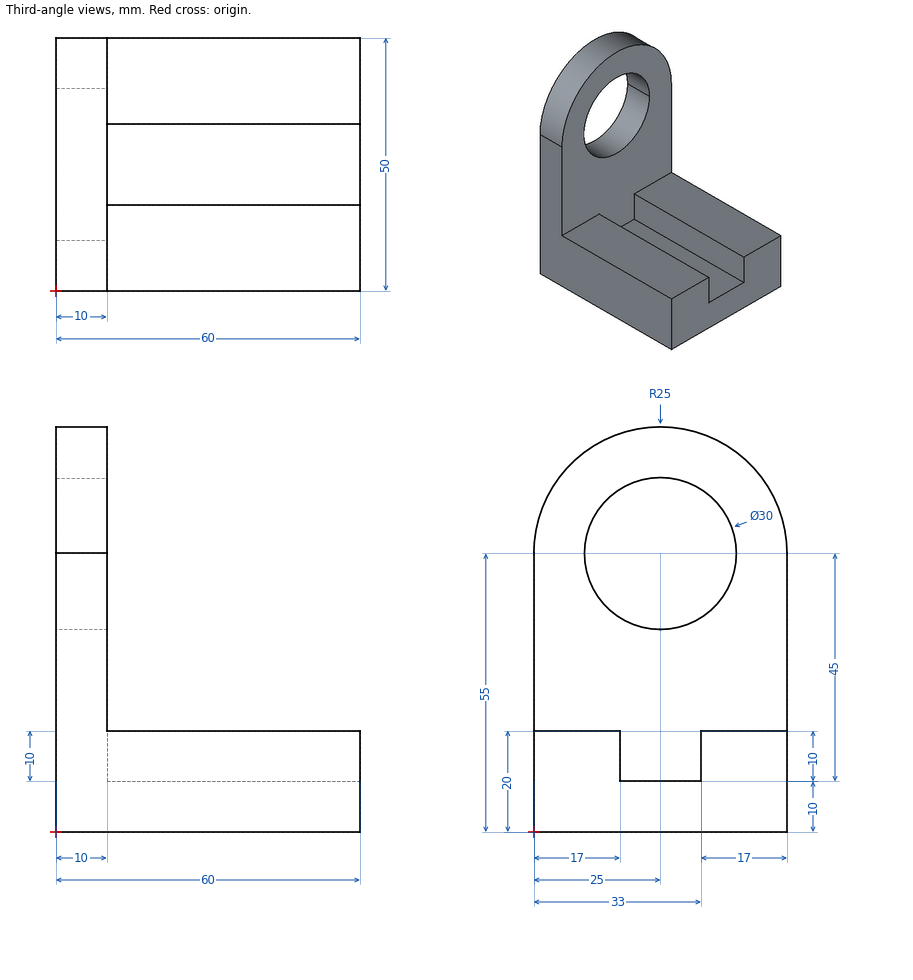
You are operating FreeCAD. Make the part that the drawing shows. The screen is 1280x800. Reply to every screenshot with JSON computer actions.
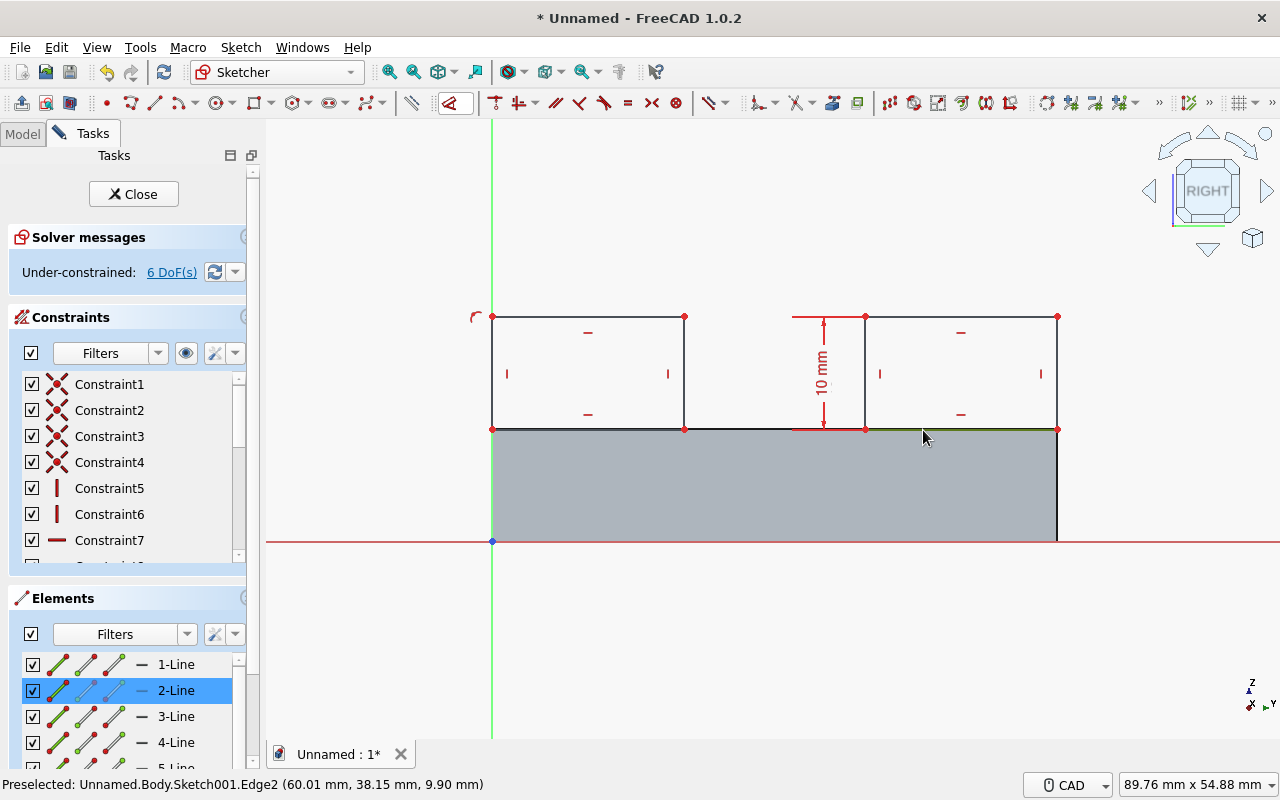
{"action": "key", "text": "l"}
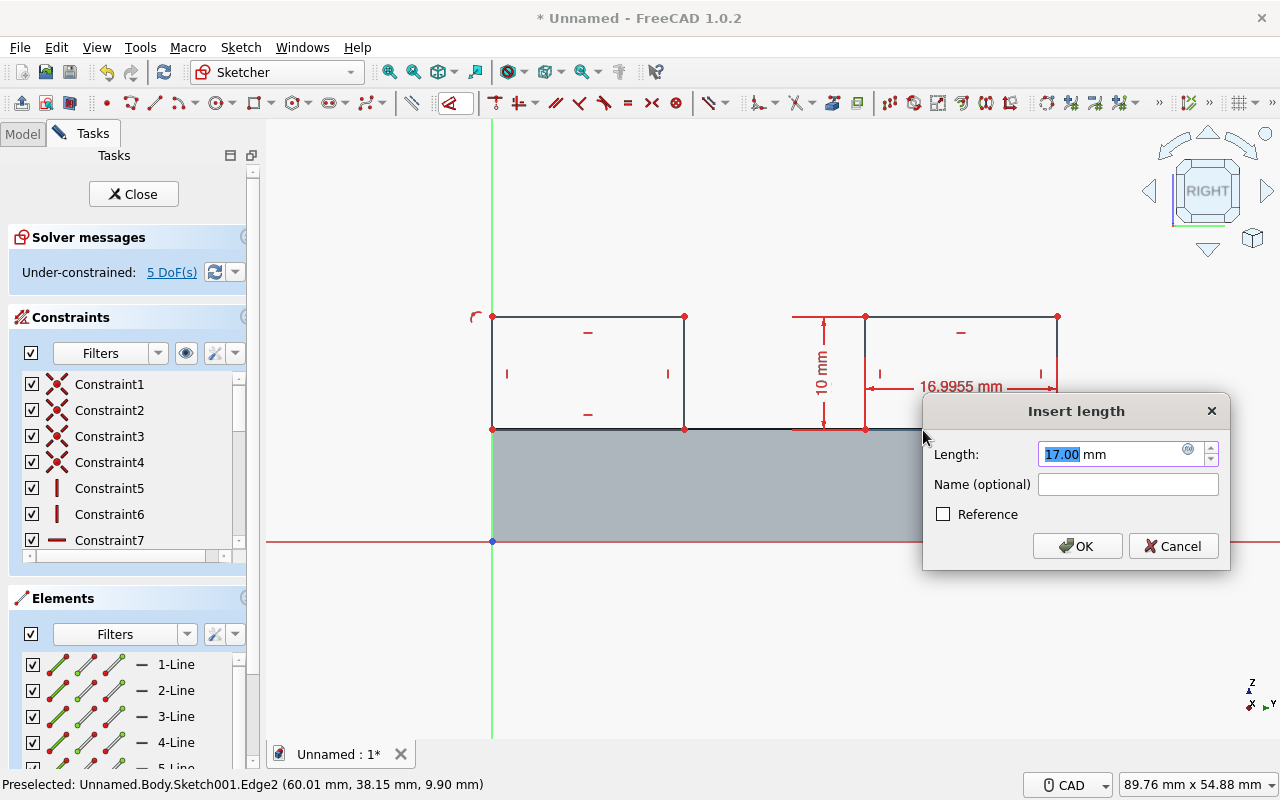
{"action": "type", "text": "17"}
{"action": "key", "text": "Return"}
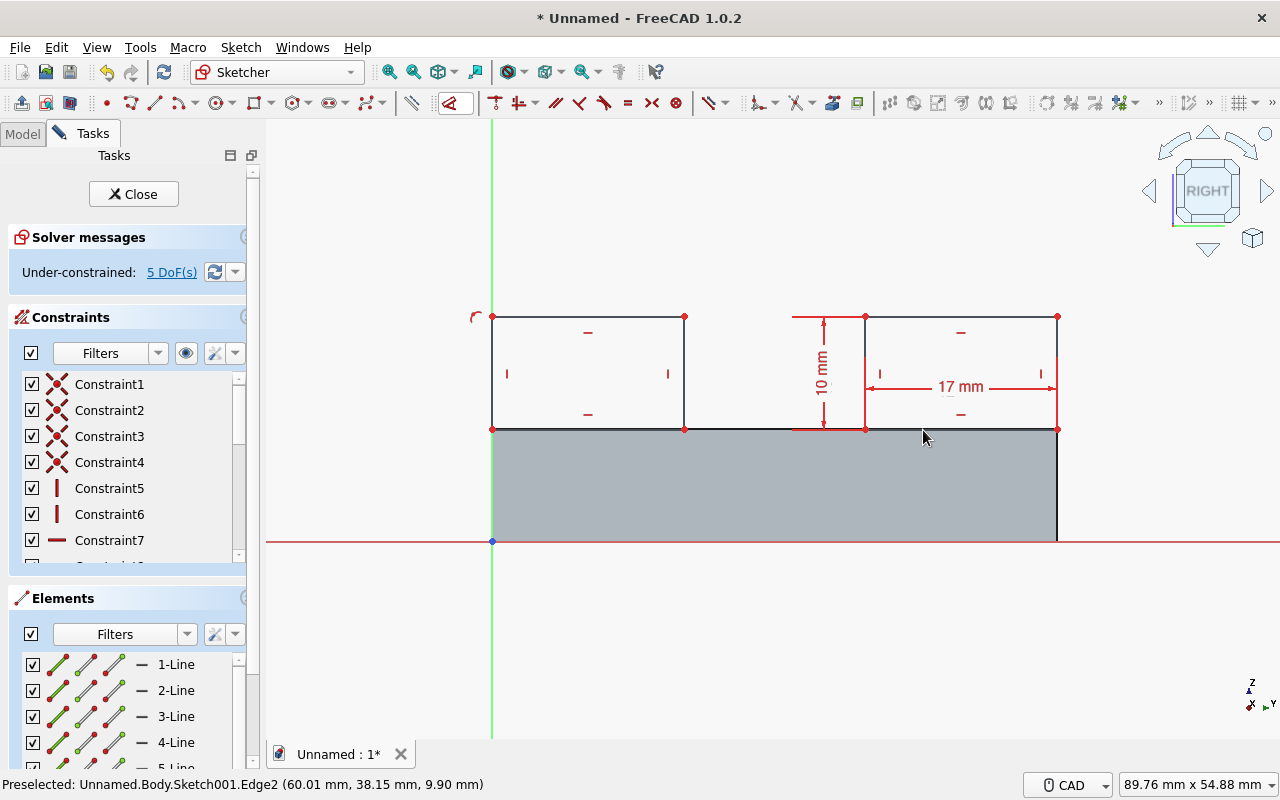
{"action": "left_click", "coordinate": [492, 351]}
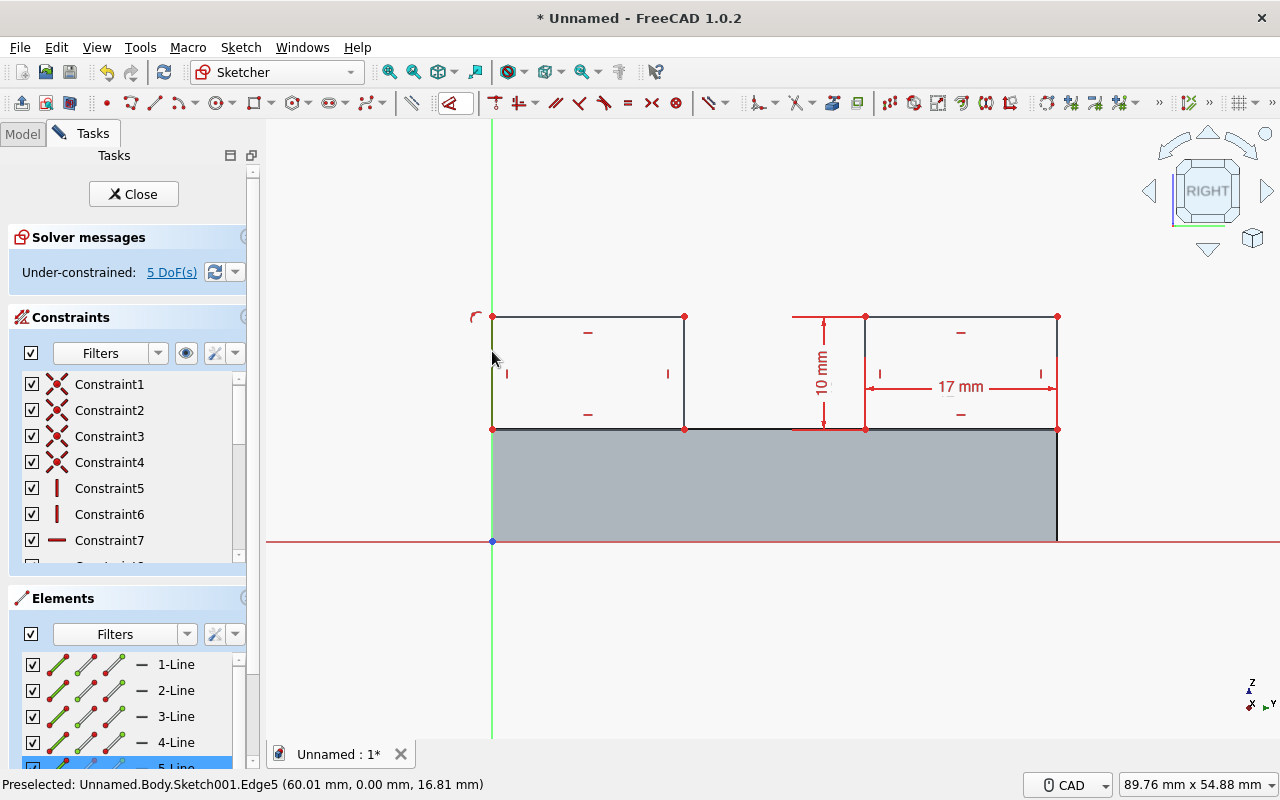
{"action": "left_click", "coordinate": [468, 104]}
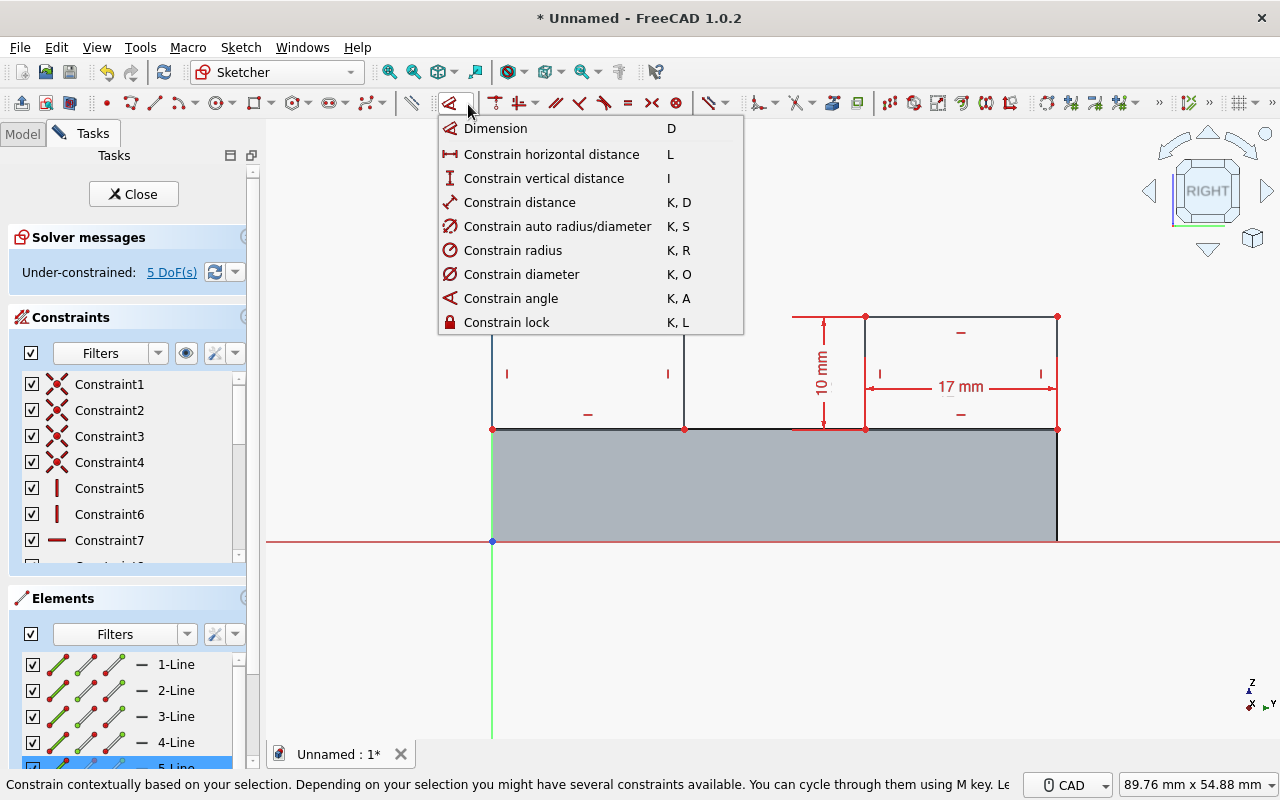
{"action": "left_click", "coordinate": [591, 178]}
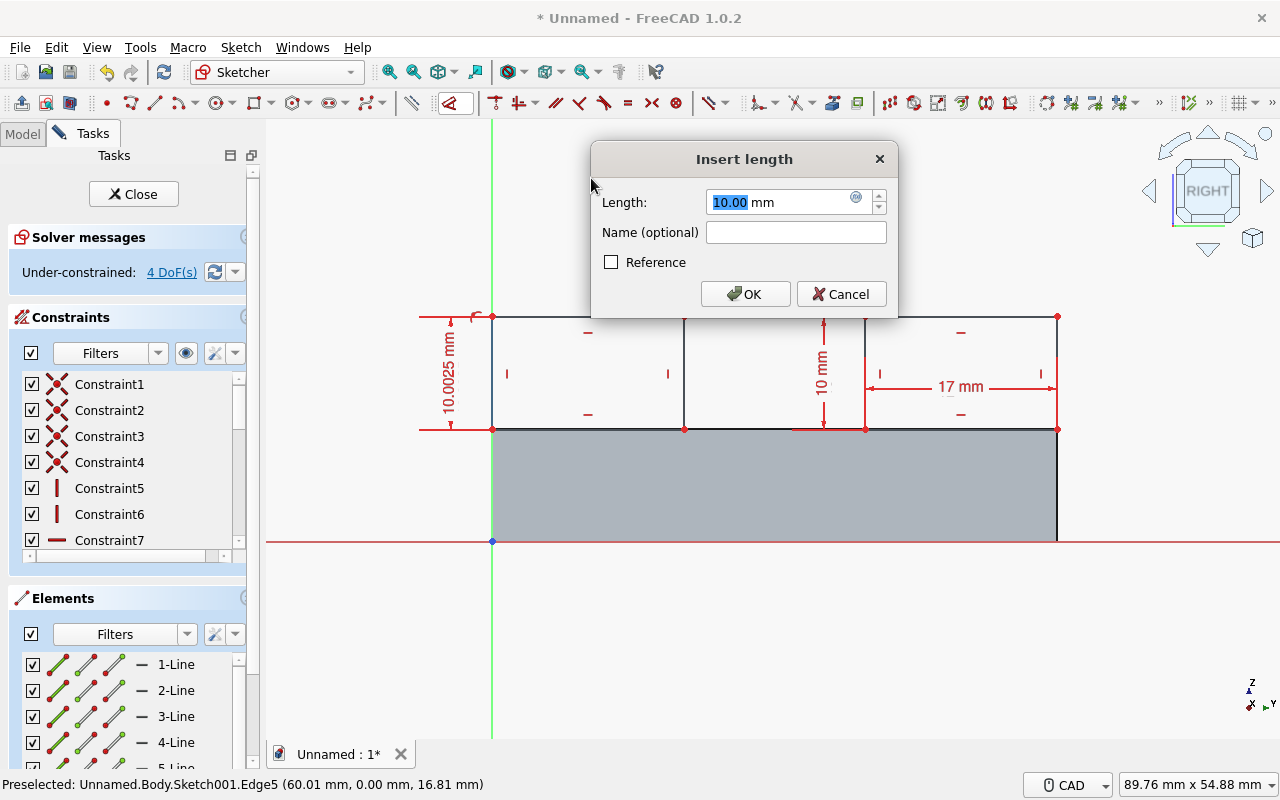
{"action": "type", "text": "10"}
{"action": "key", "text": "Return"}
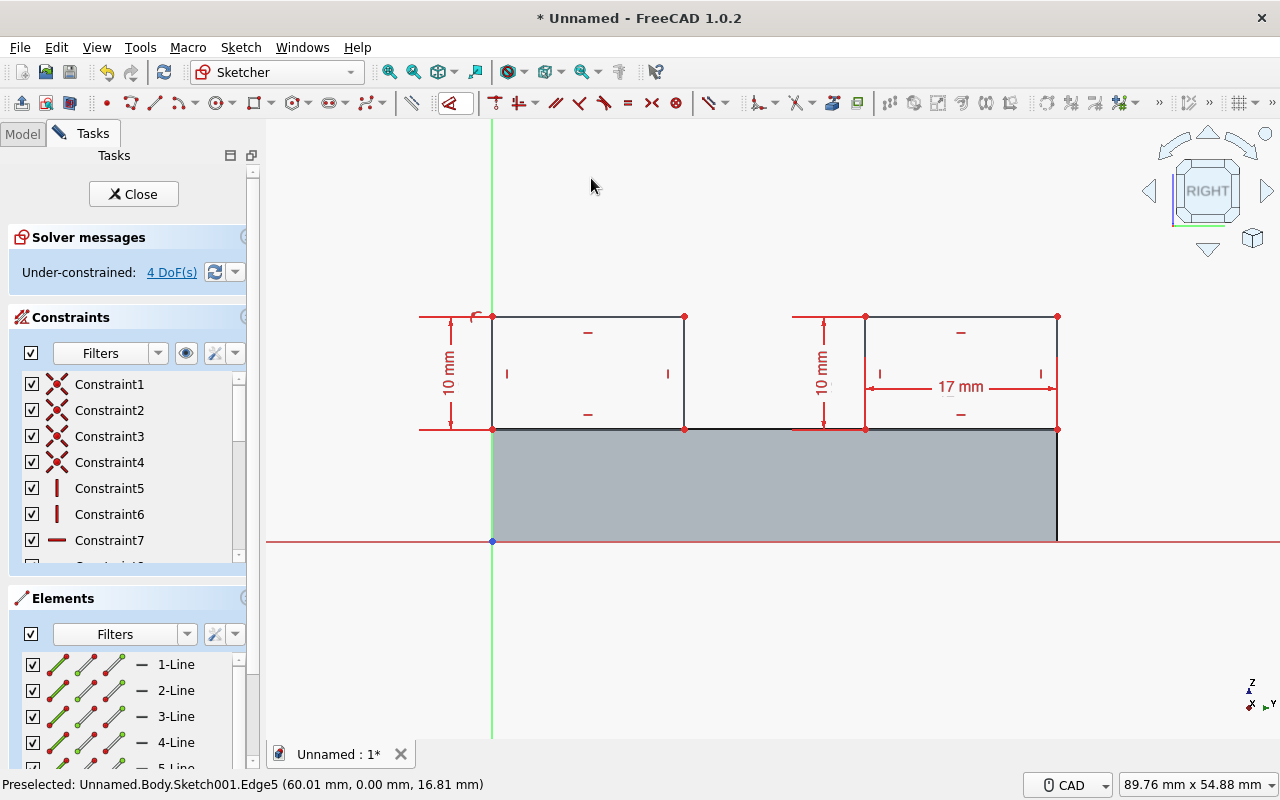
{"action": "left_click", "coordinate": [550, 430]}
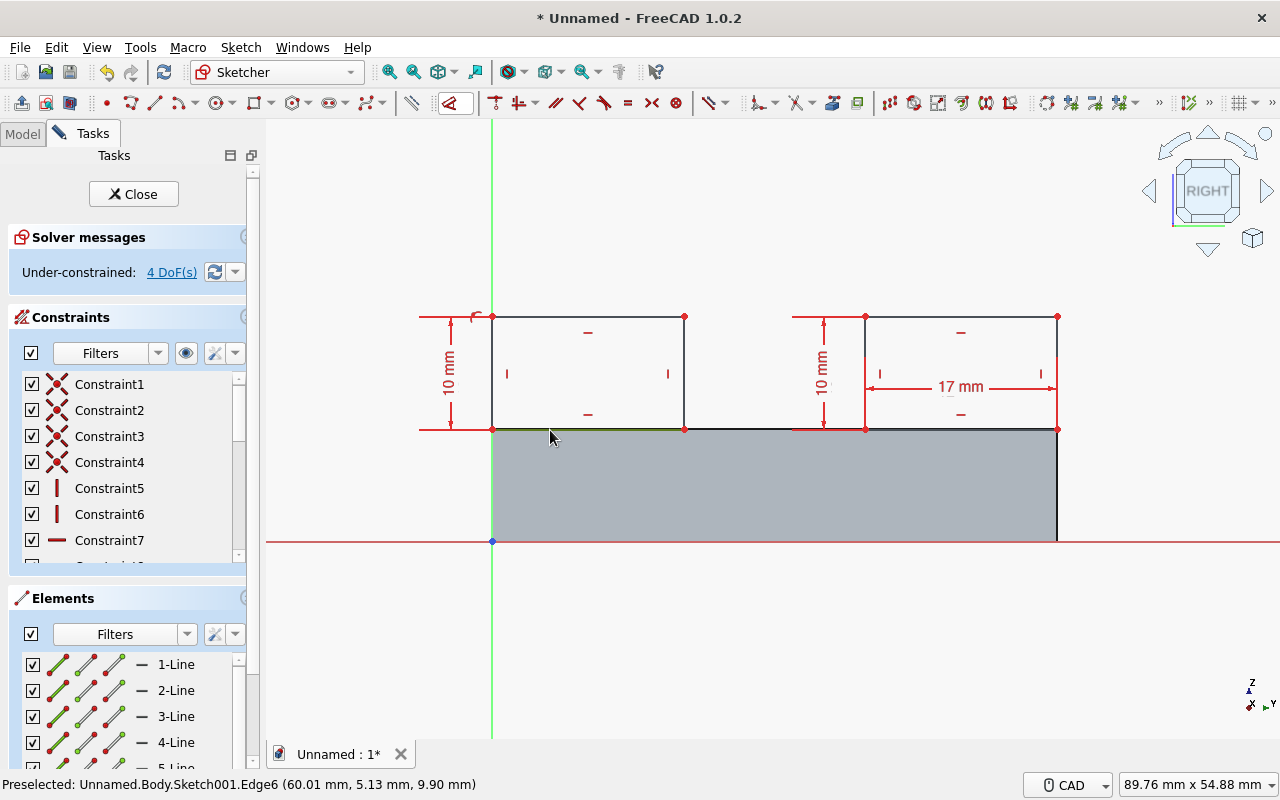
{"action": "key", "text": "l"}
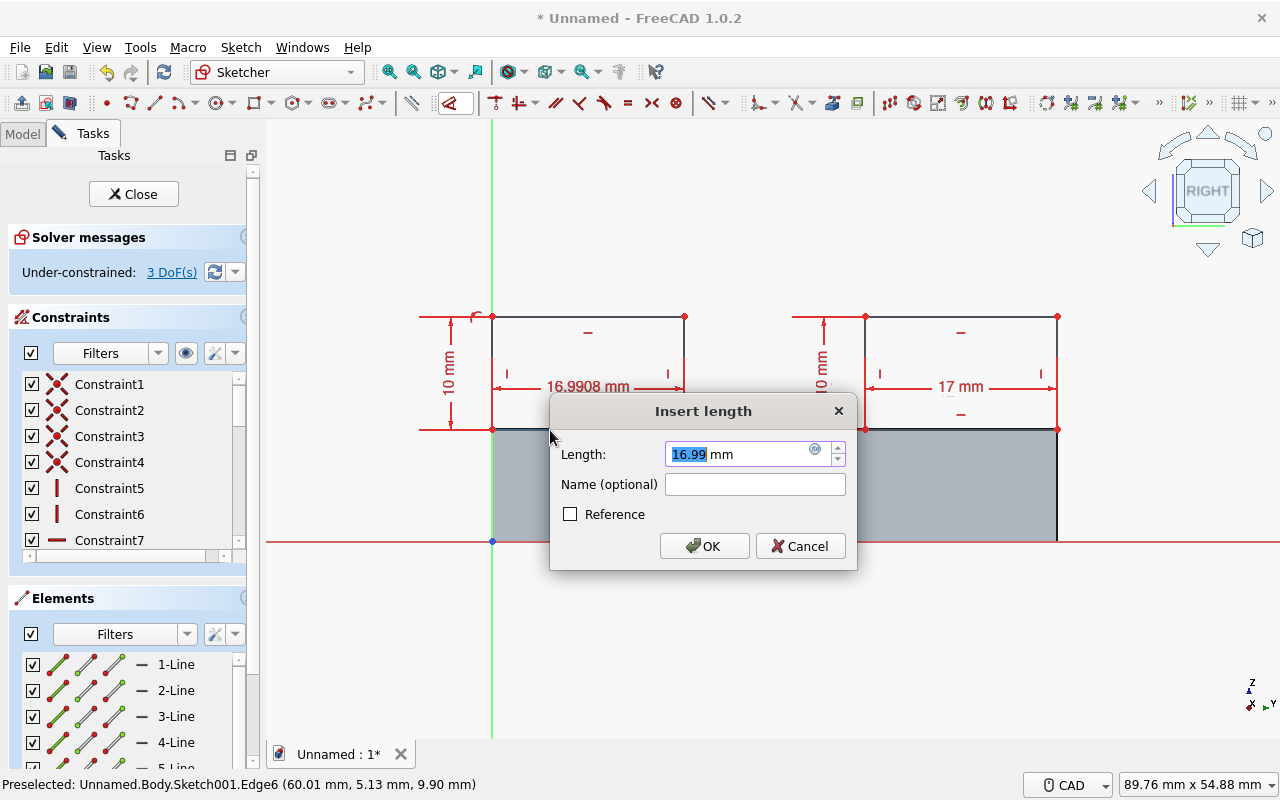
{"action": "type", "text": "17"}
{"action": "key", "text": "Return"}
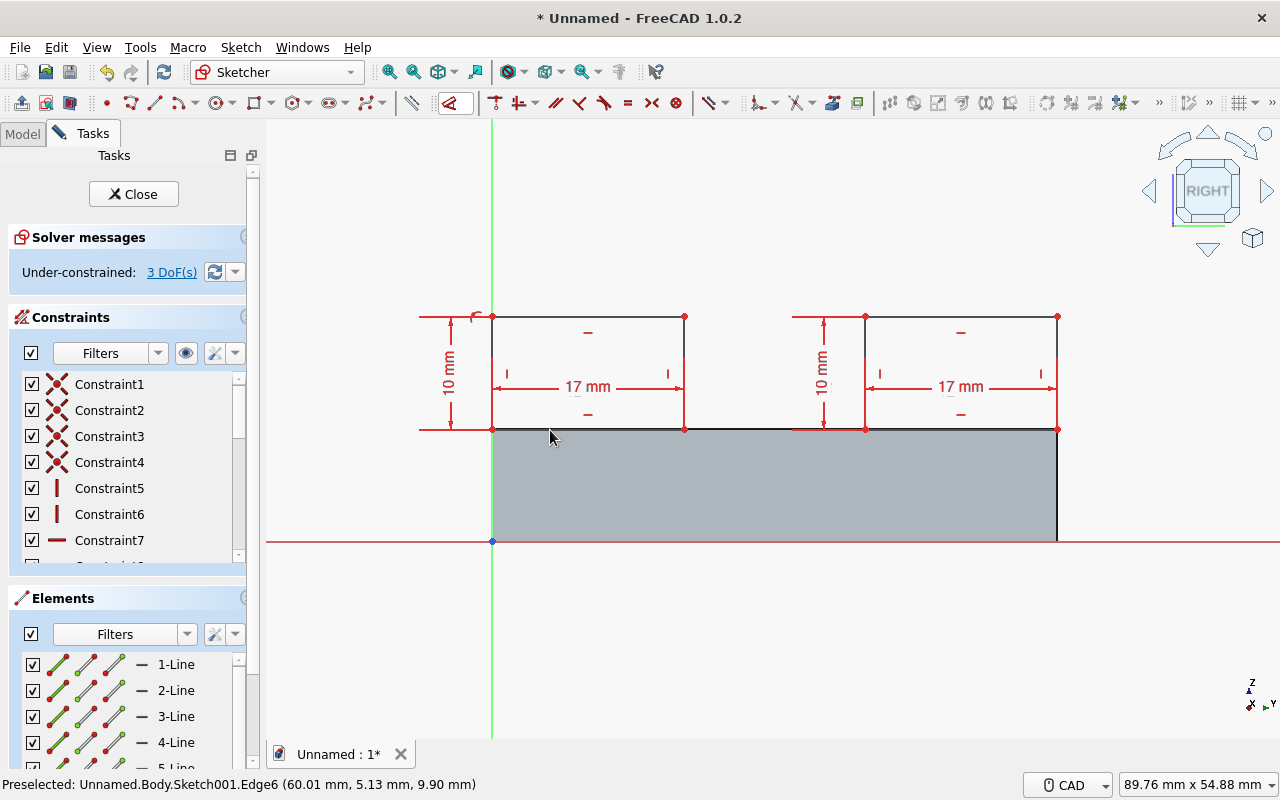
{"action": "left_click", "coordinate": [865, 317]}